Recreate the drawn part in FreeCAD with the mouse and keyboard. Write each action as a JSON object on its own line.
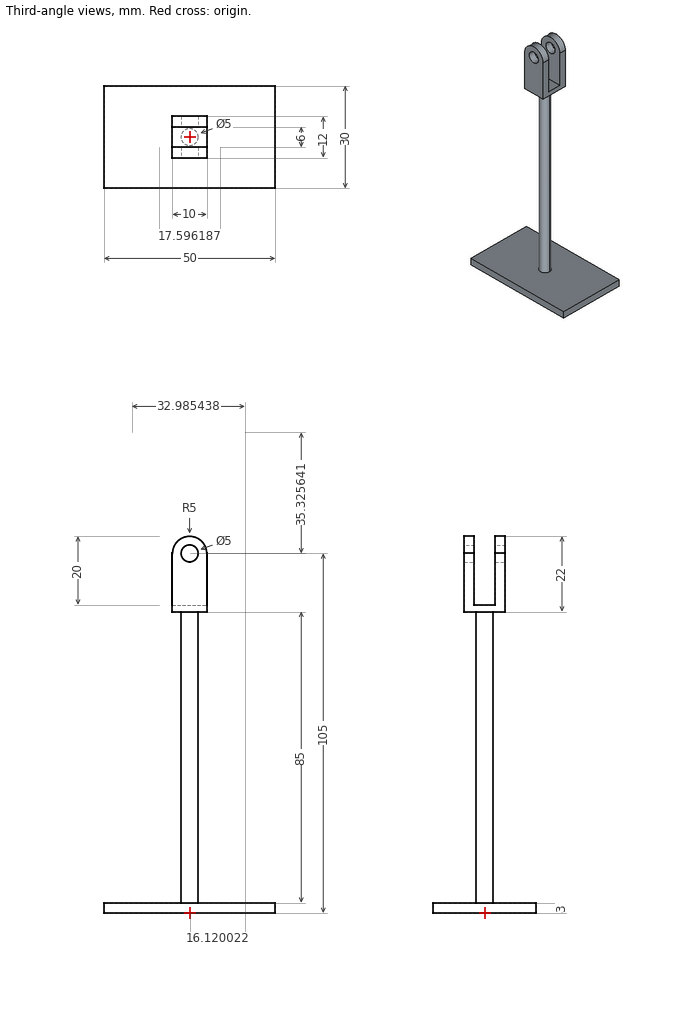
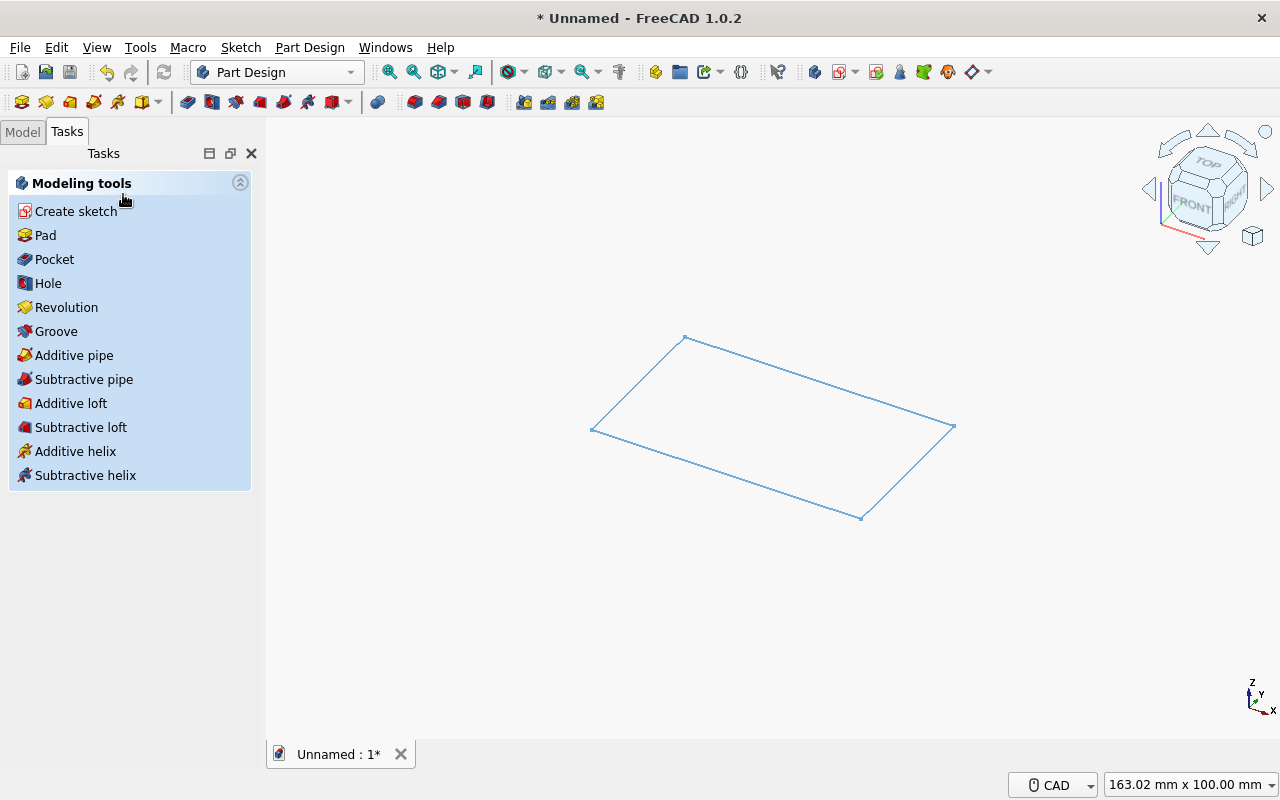
{"action": "left_click", "coordinate": [22, 102]}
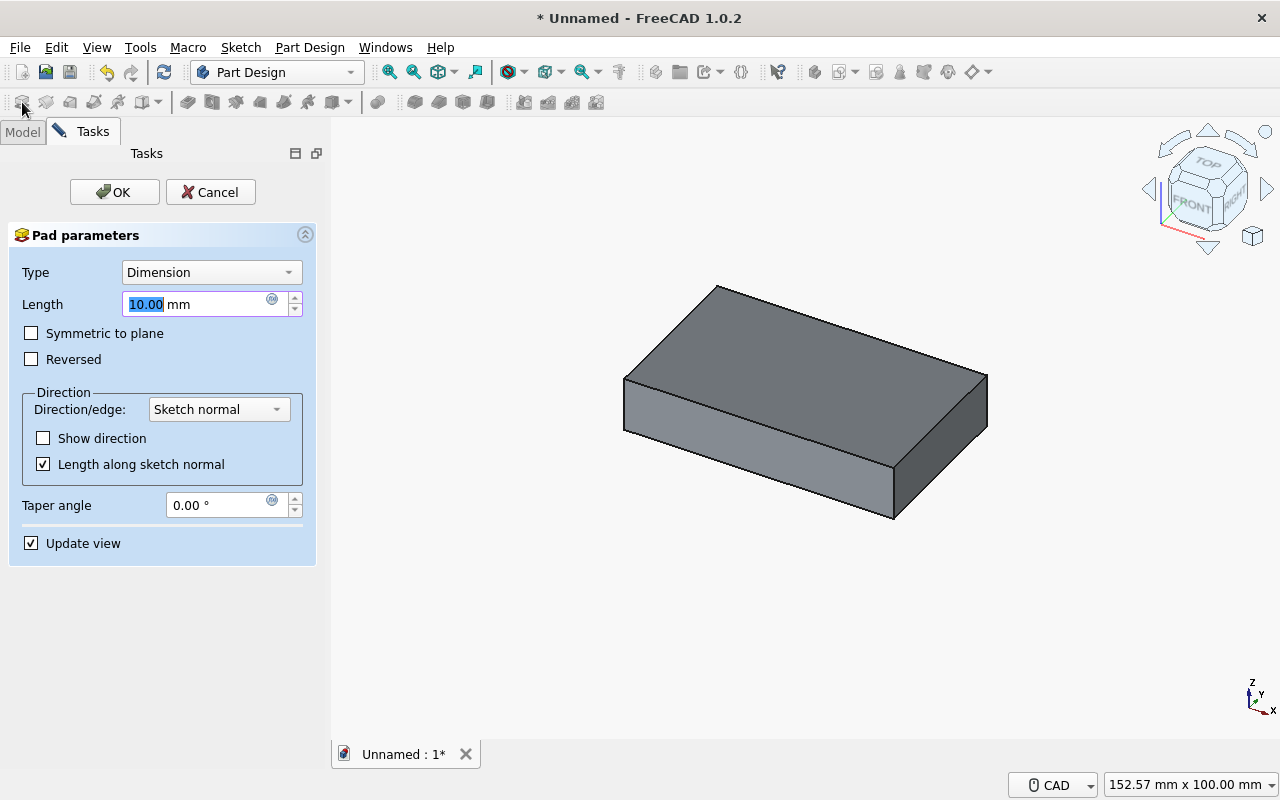
{"action": "type", "text": "3"}
{"action": "key", "text": "Tab"}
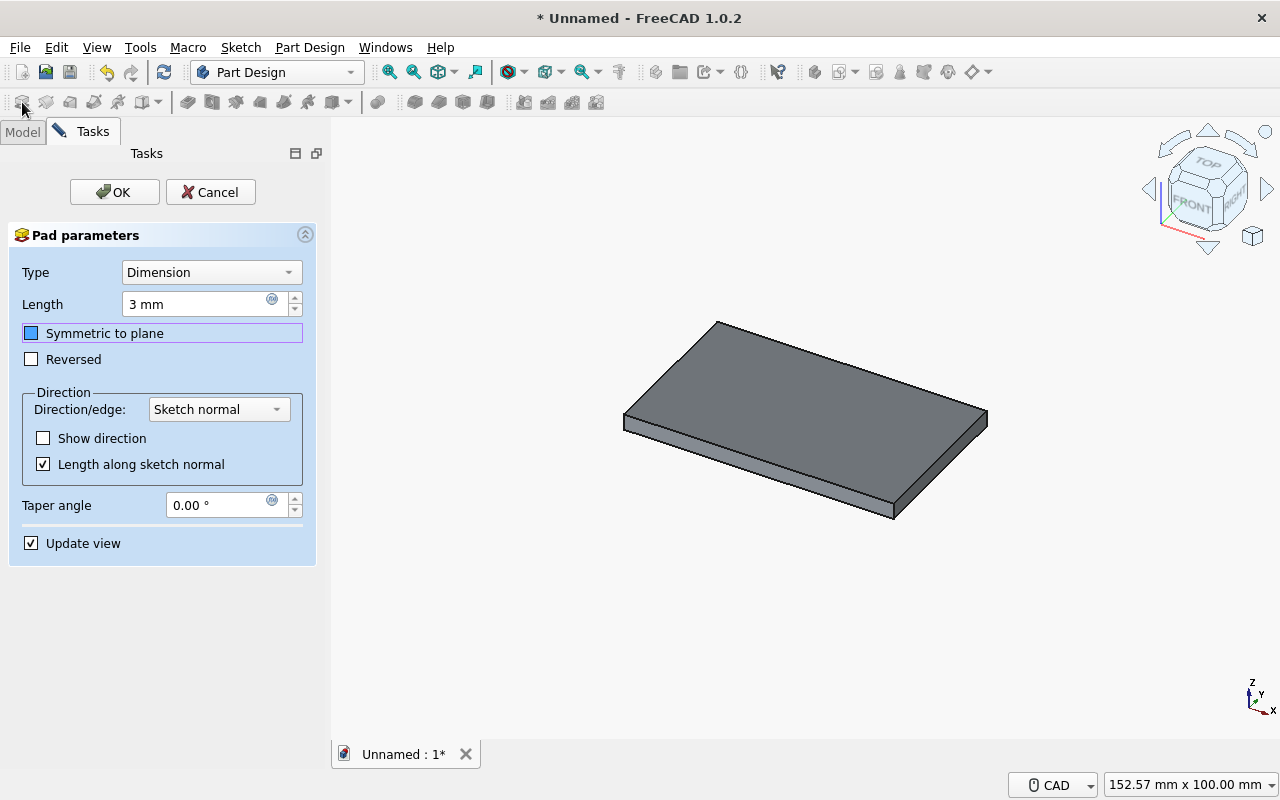
{"action": "left_click", "coordinate": [115, 192]}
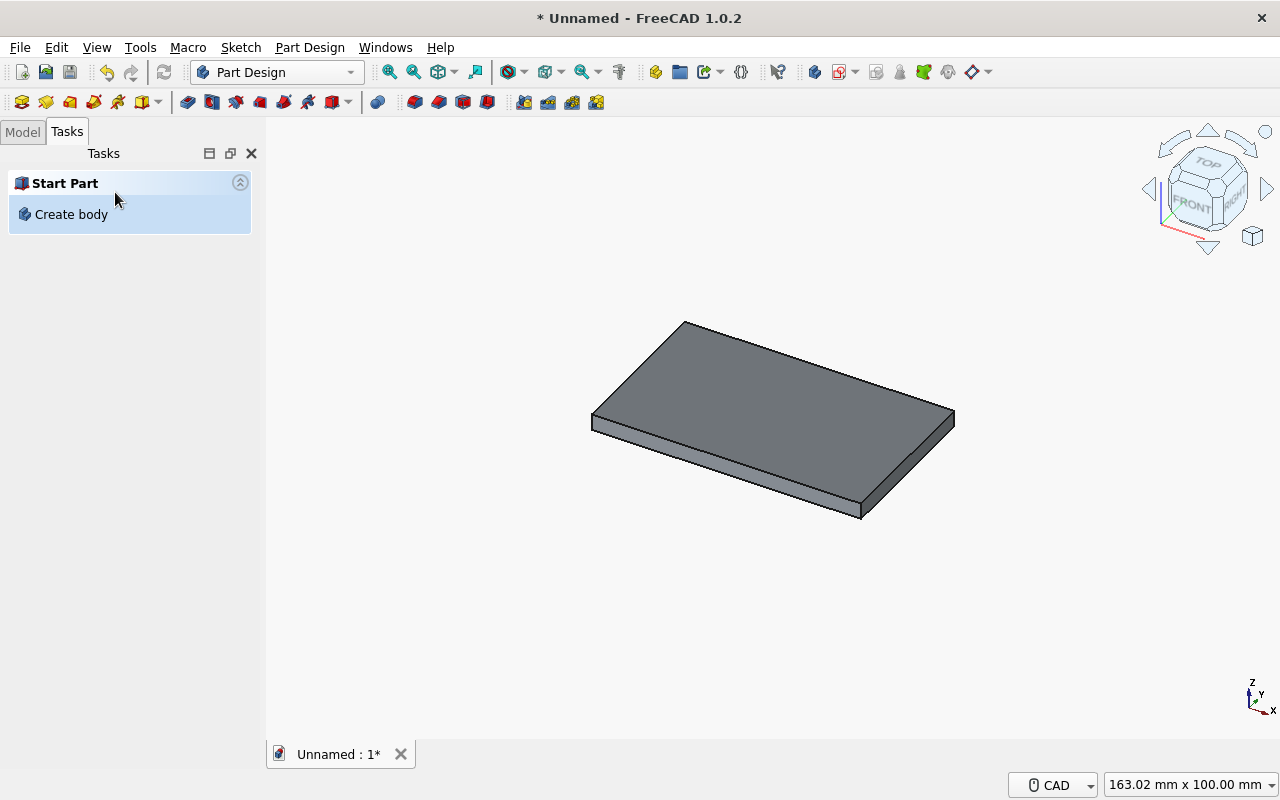
{"action": "left_click", "coordinate": [390, 72]}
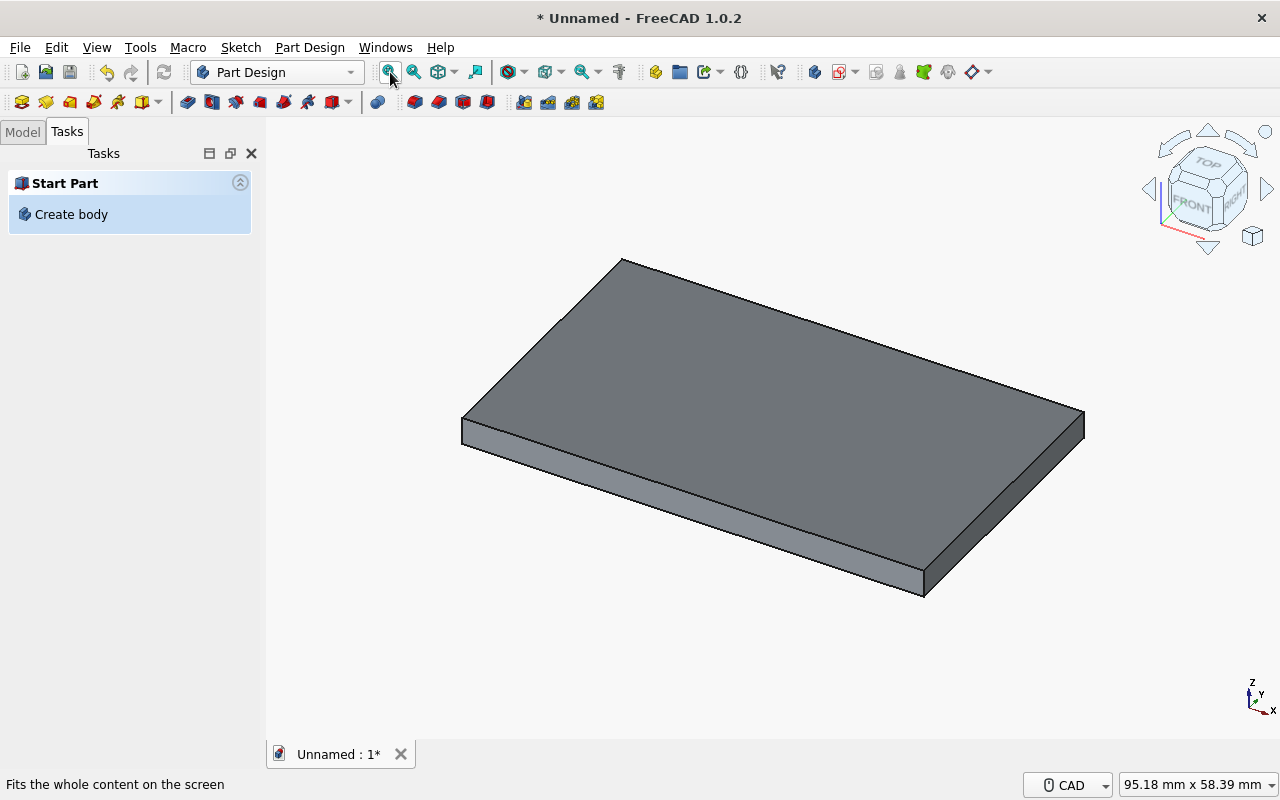
{"action": "left_click", "coordinate": [839, 436]}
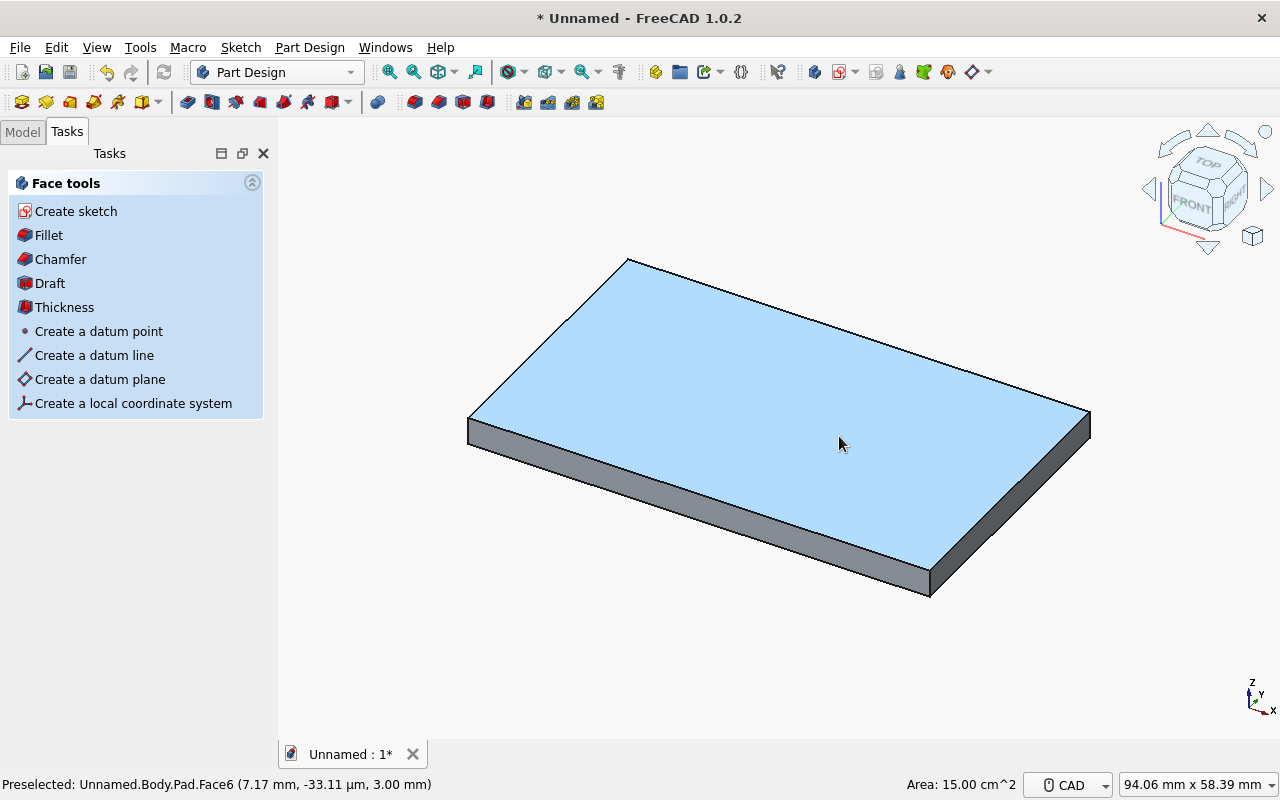
{"action": "left_click", "coordinate": [840, 72]}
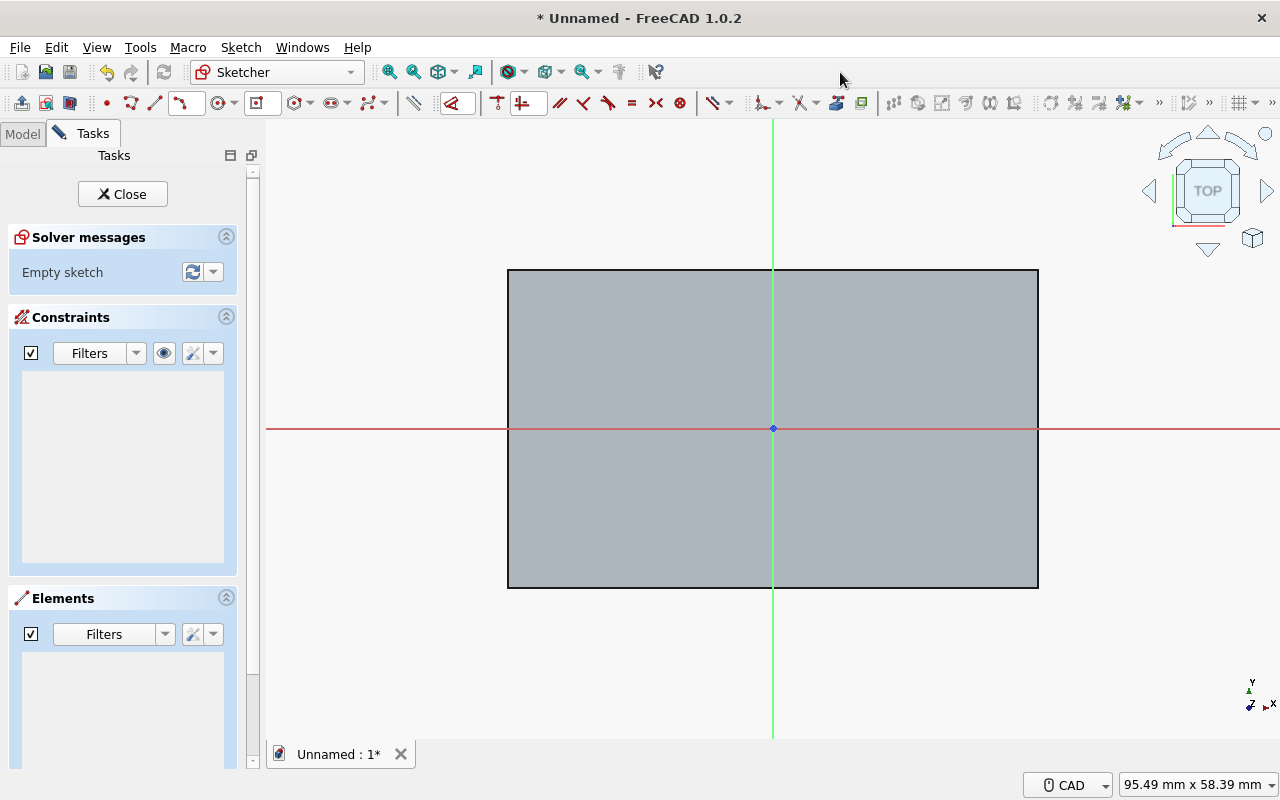
{"action": "scroll", "coordinate": [784, 429], "scroll_direction": "up", "scroll_amount": 10}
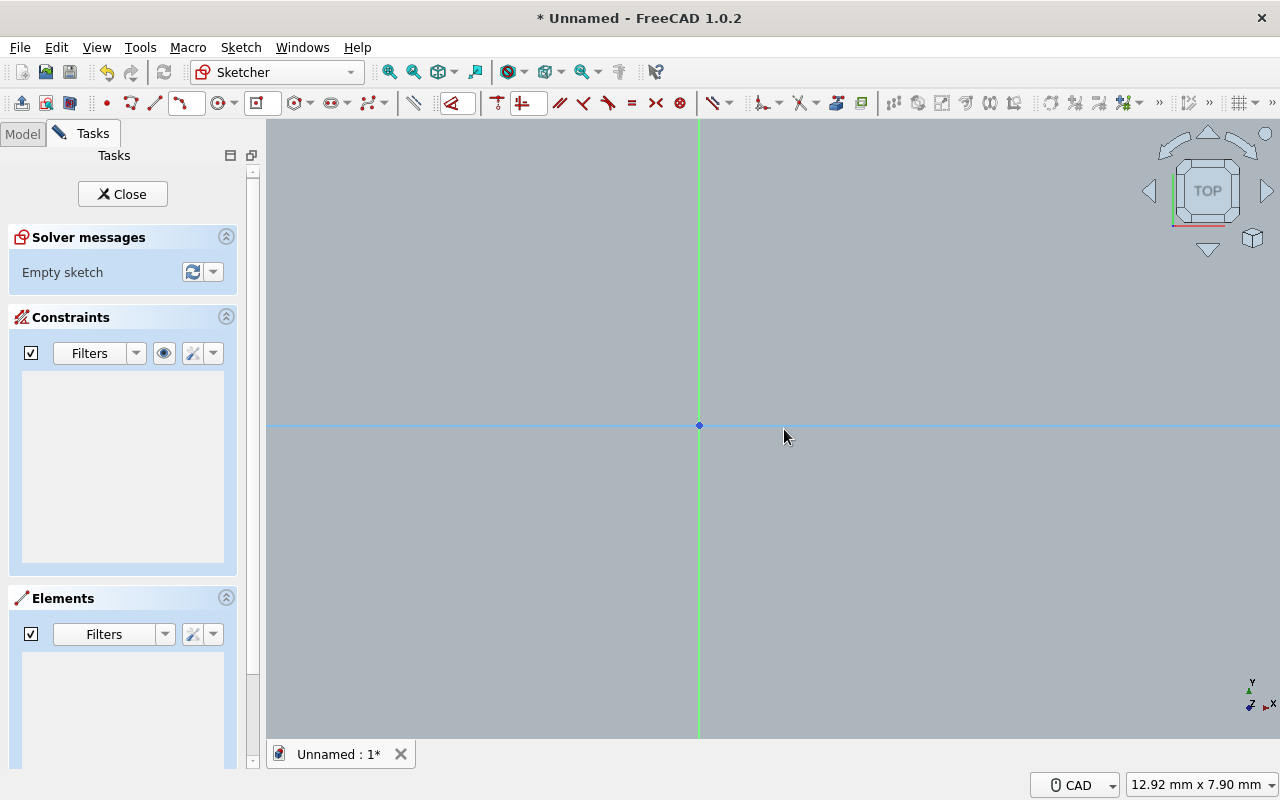
{"action": "left_click", "coordinate": [218, 104]}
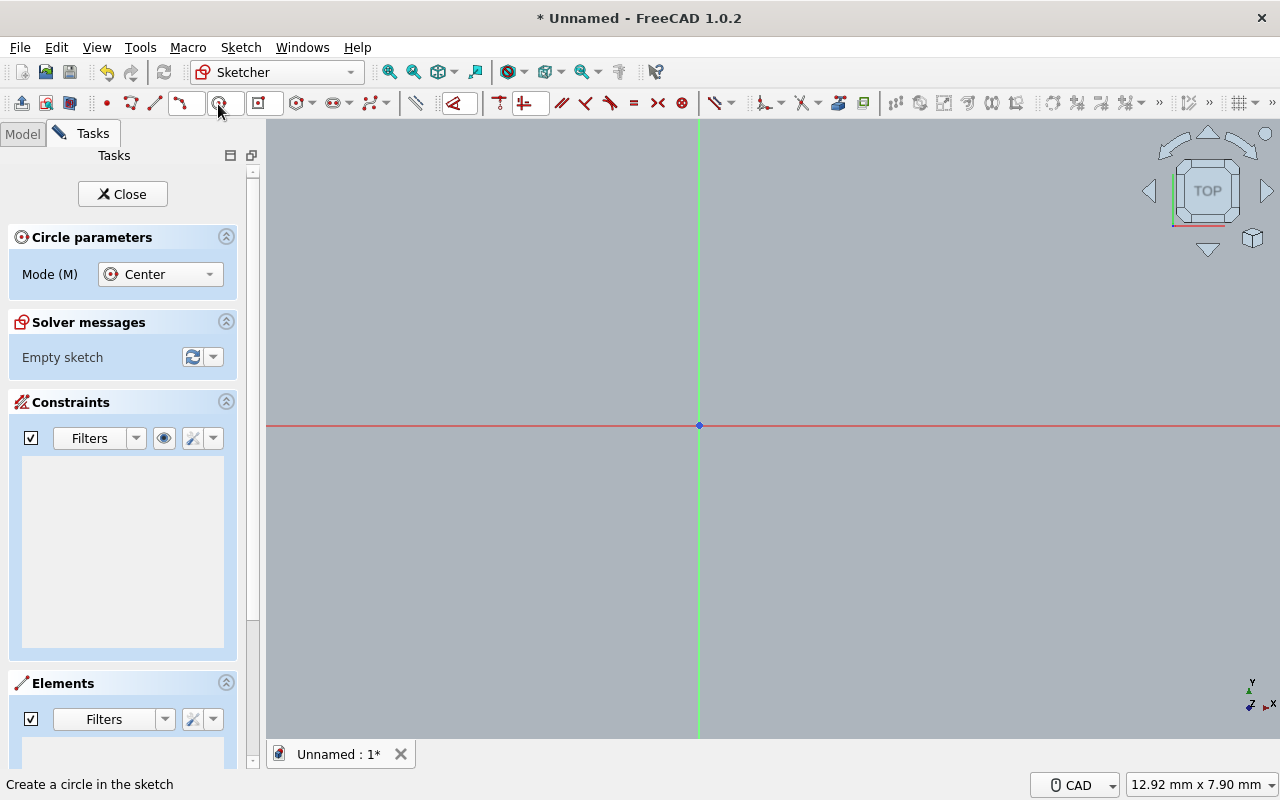
{"action": "left_click", "coordinate": [699, 426]}
{"action": "mouse_move", "coordinate": [838, 287]}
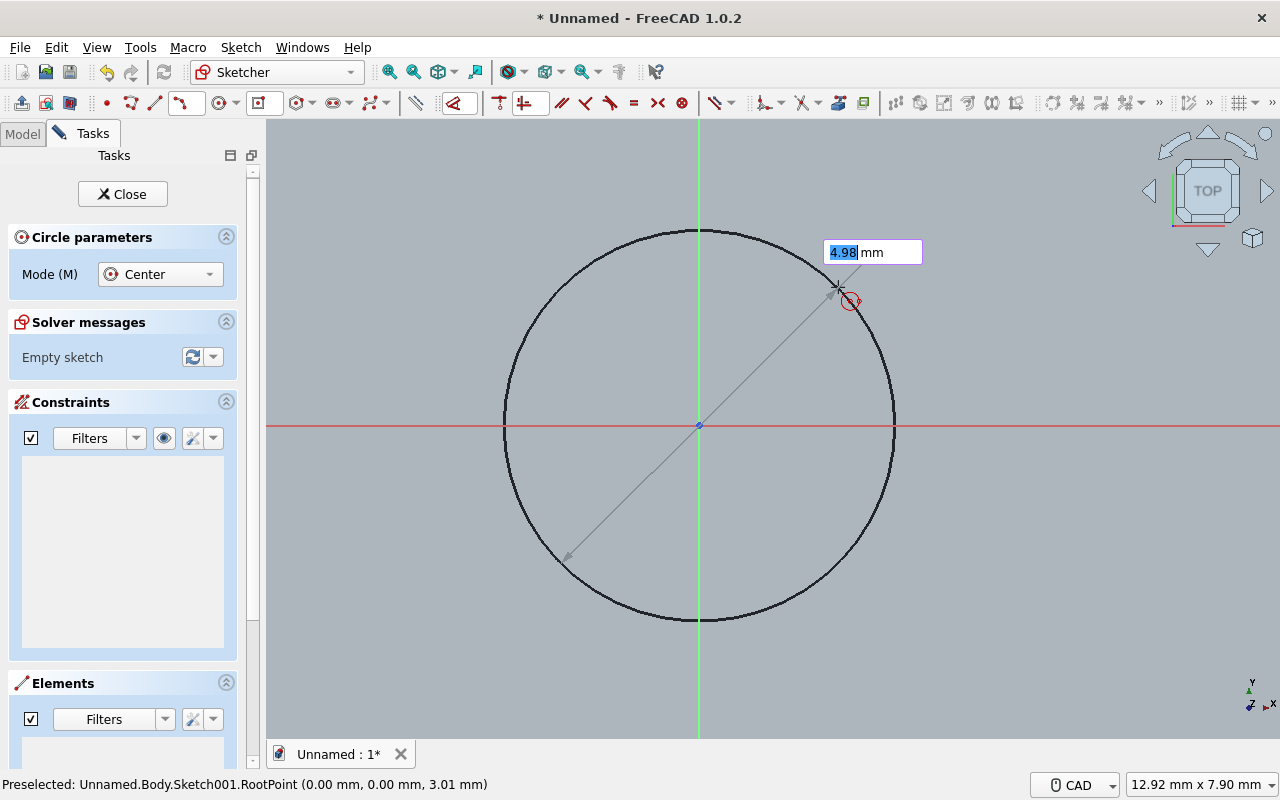
{"action": "type", "text": "5"}
{"action": "key", "text": "Return"}
{"action": "key", "text": "Escape"}